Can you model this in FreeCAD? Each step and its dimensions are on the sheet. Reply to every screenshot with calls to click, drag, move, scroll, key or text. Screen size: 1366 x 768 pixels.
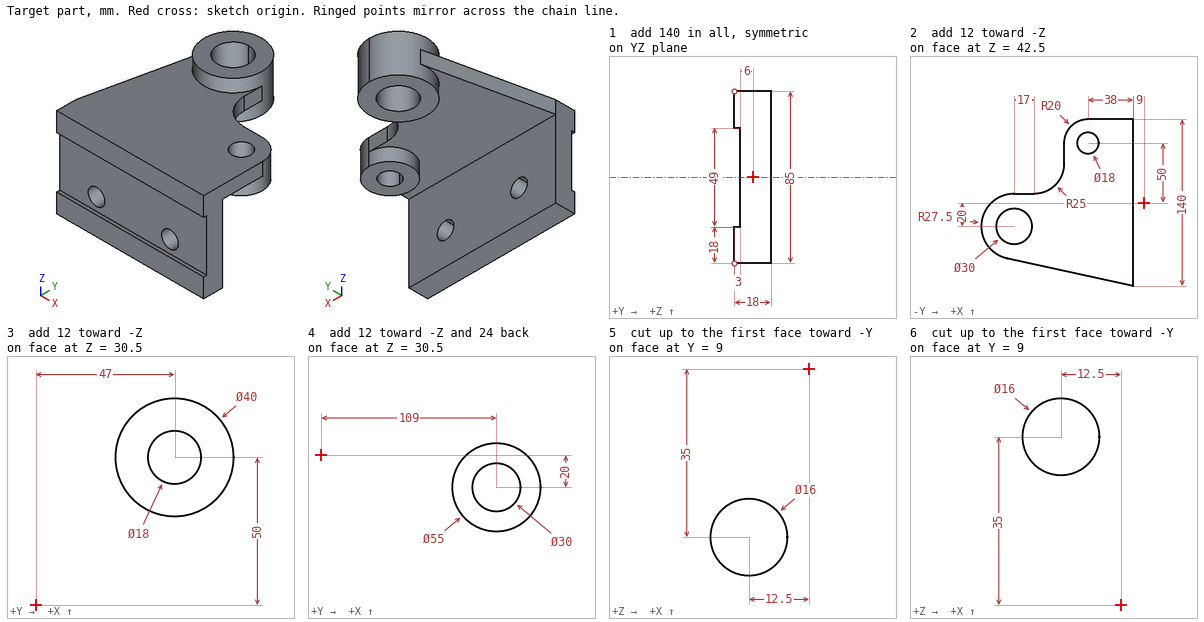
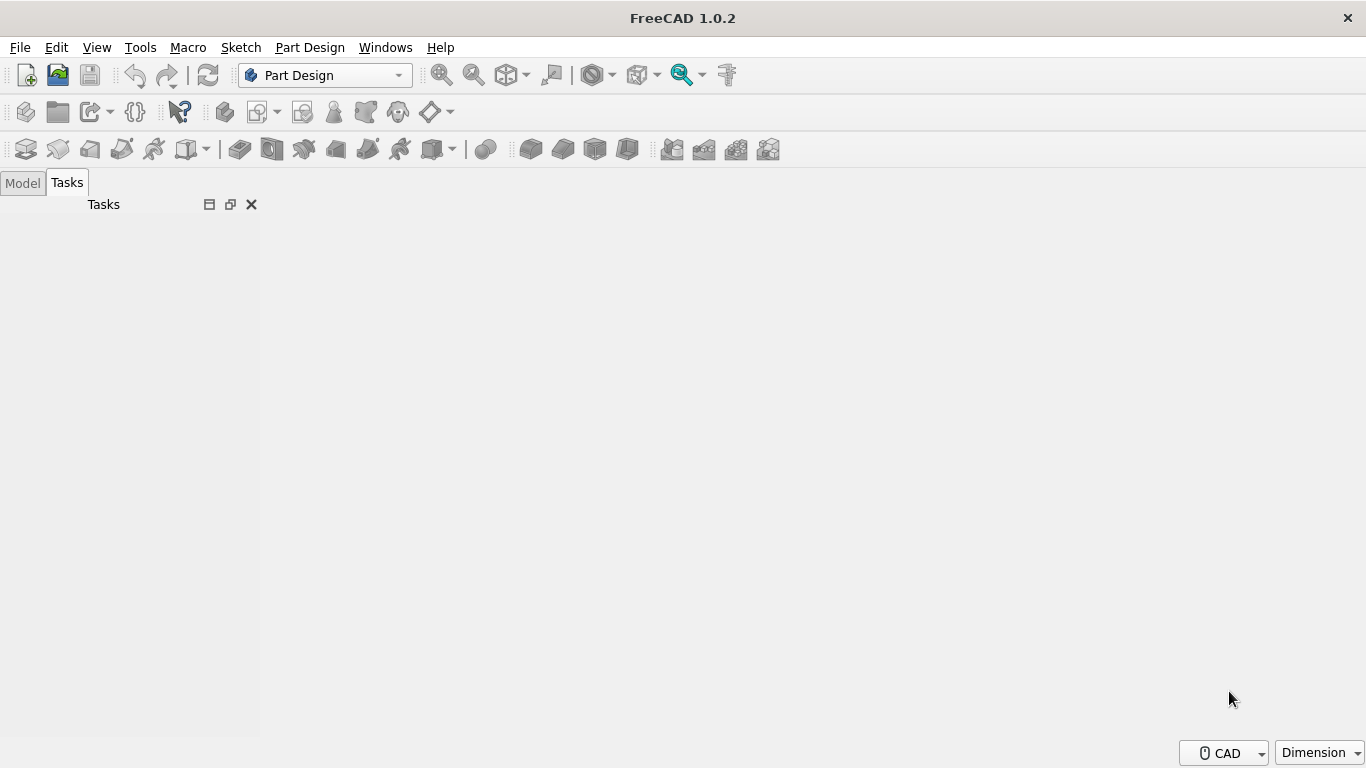
key(ctrl+n)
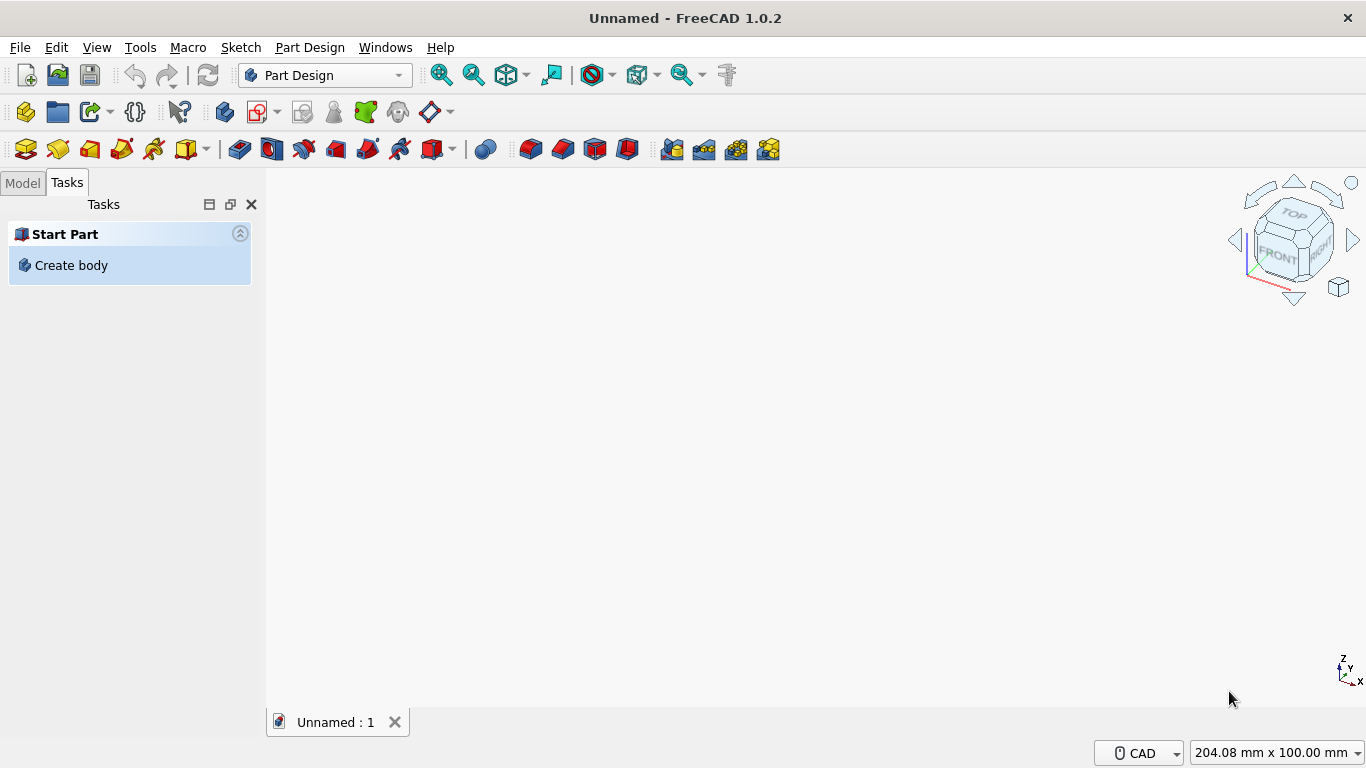
click(258, 112)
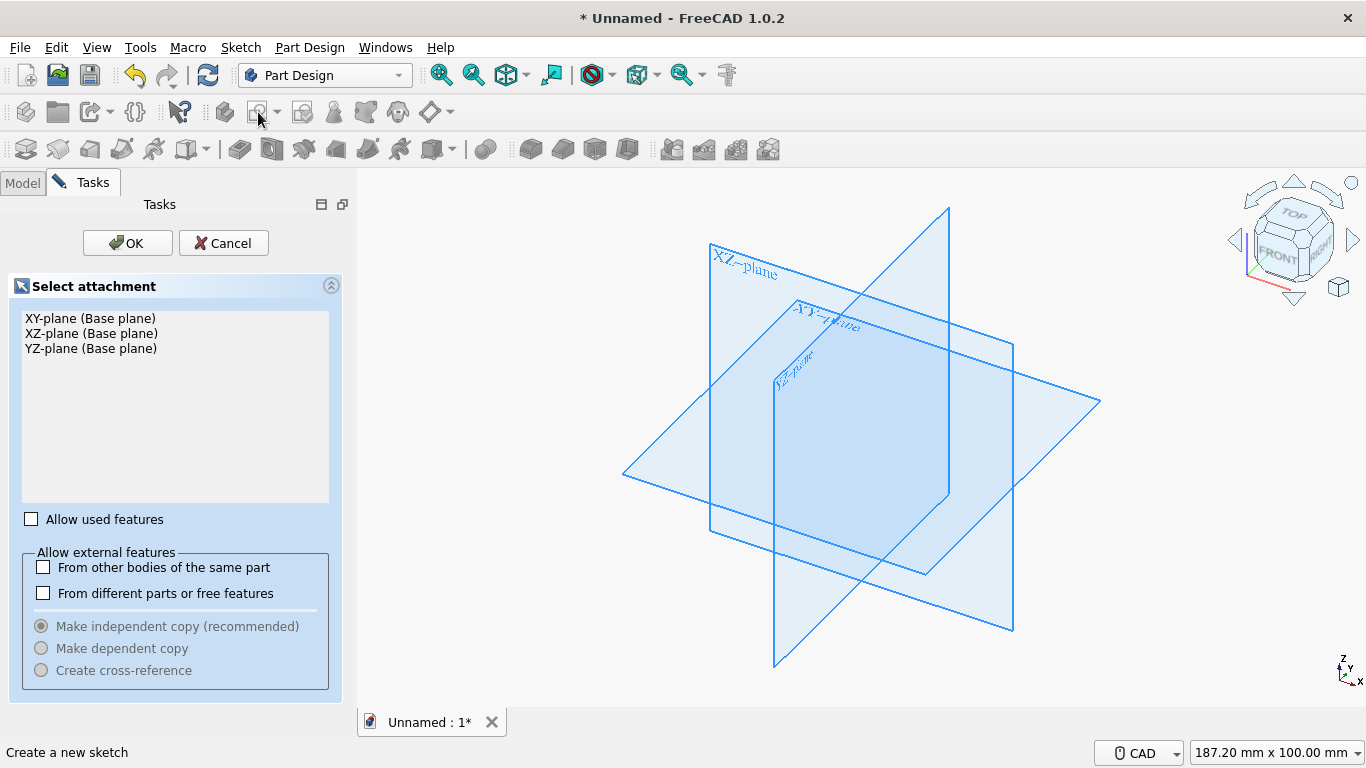
click(82, 348)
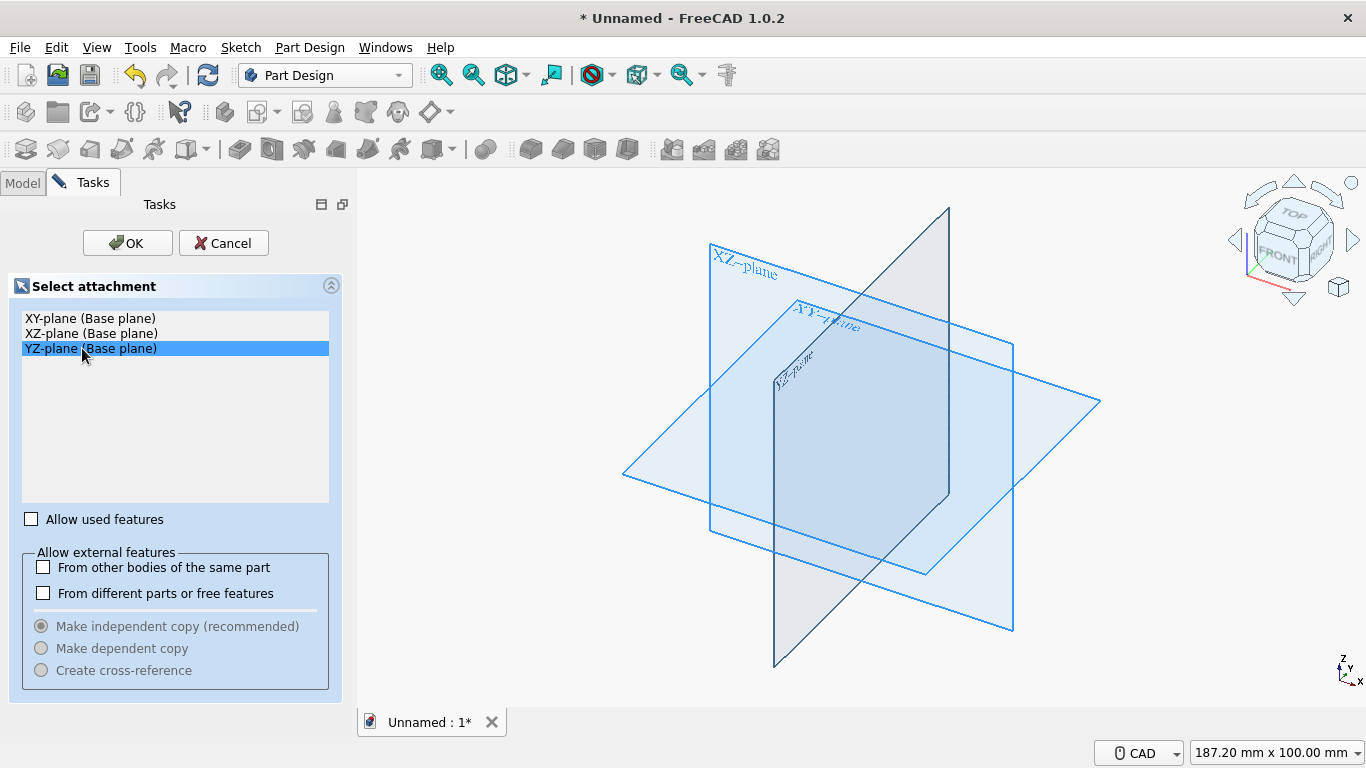
click(128, 243)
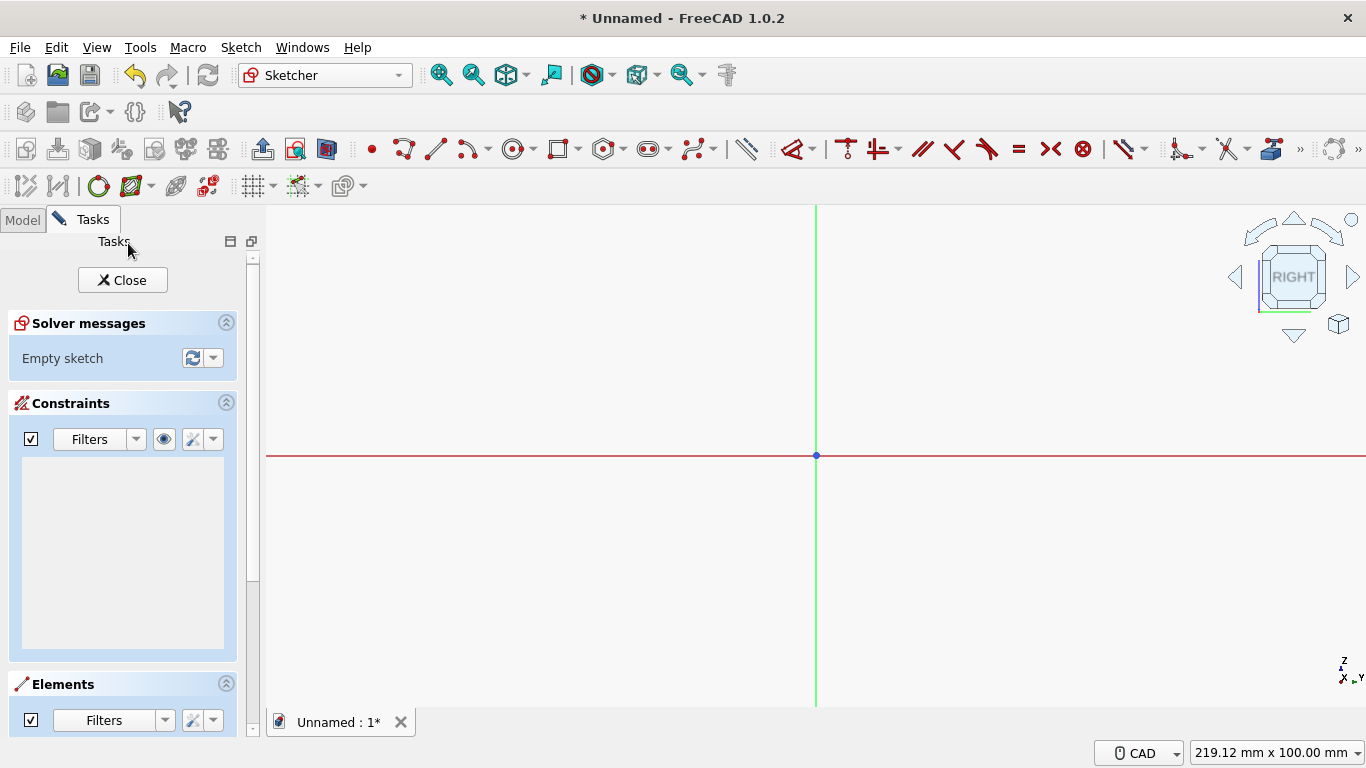
scroll(608, 456, down, 2)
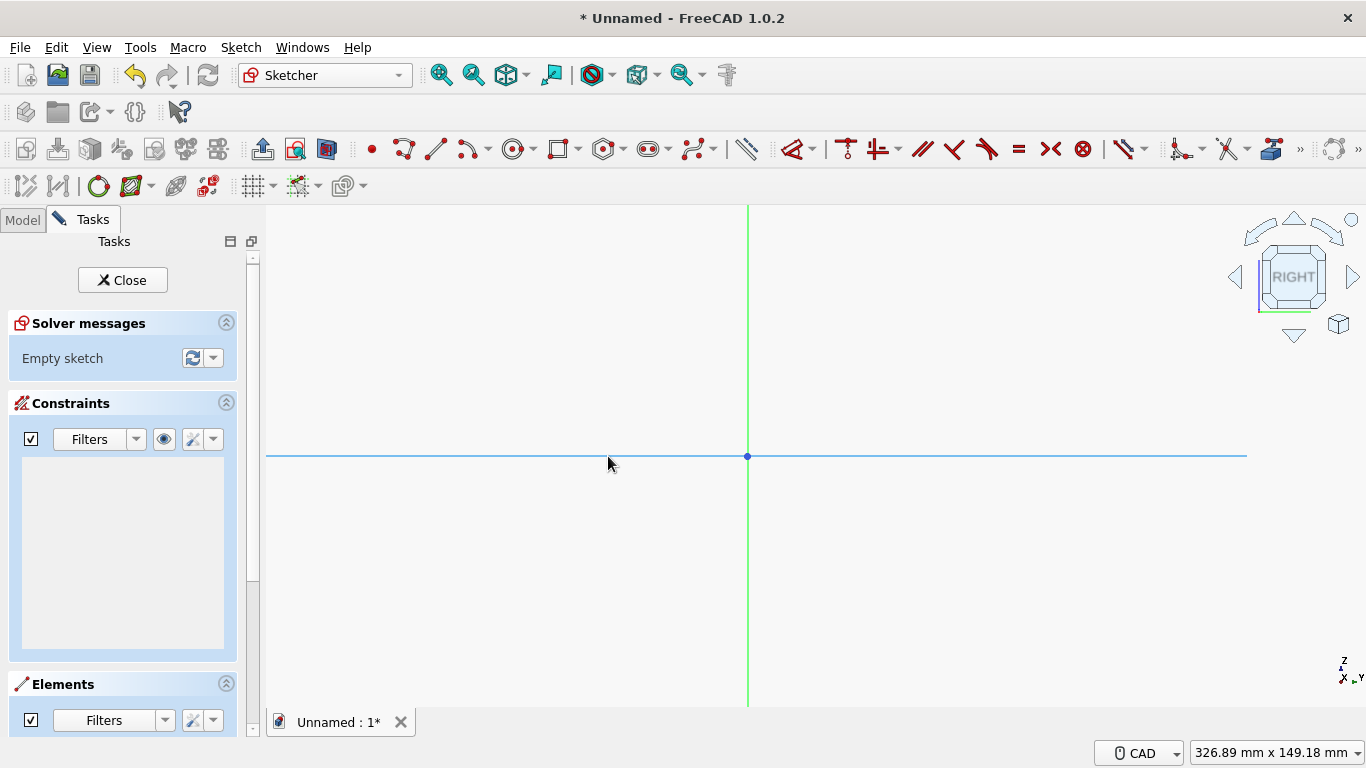
key(g)
key(m)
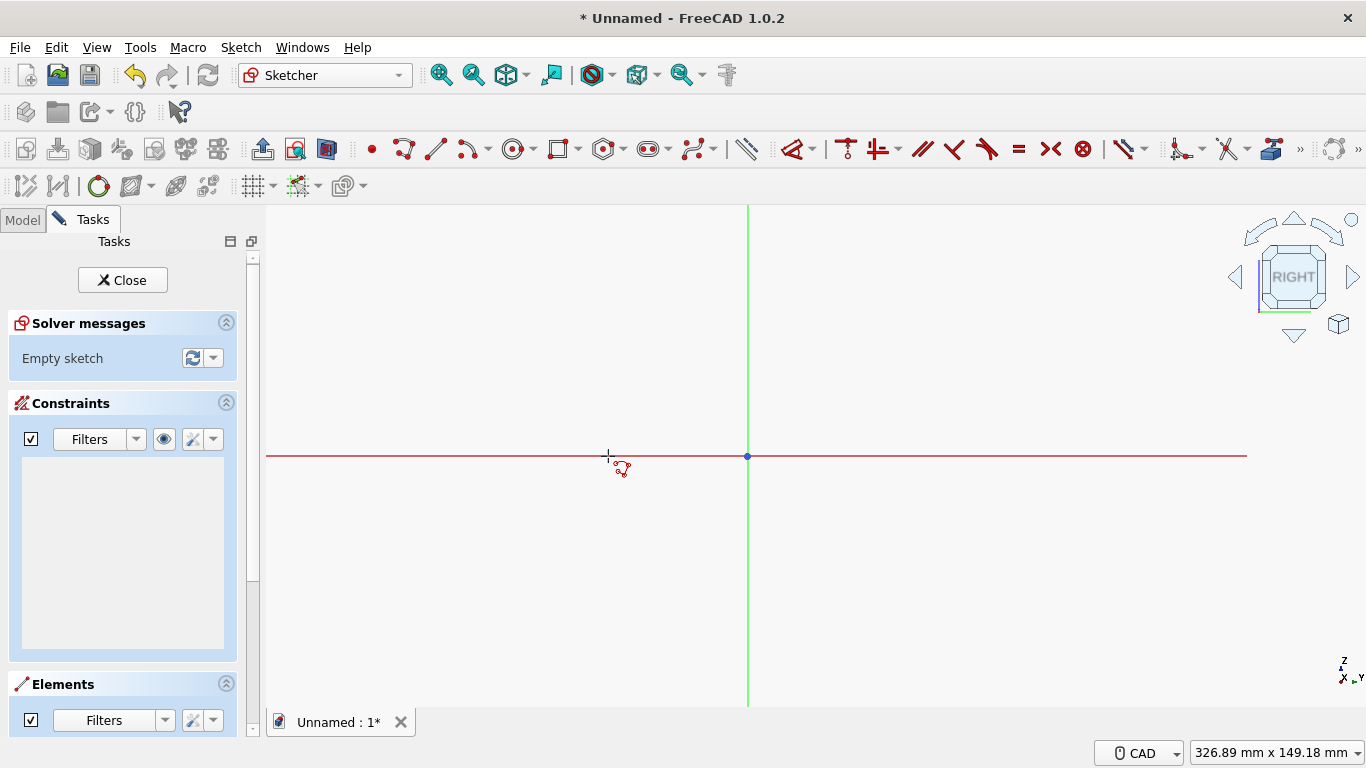
click(727, 374)
click(727, 539)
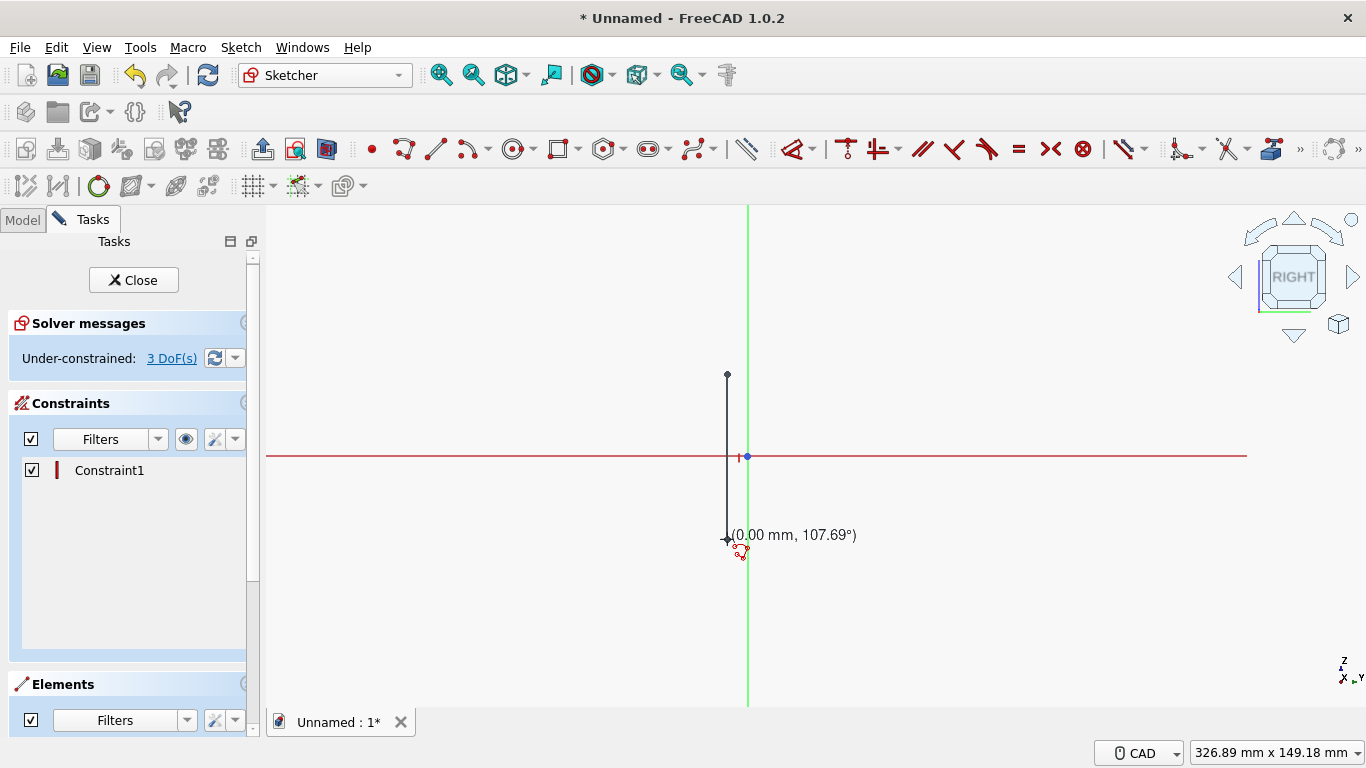
scroll(717, 539, up, 3)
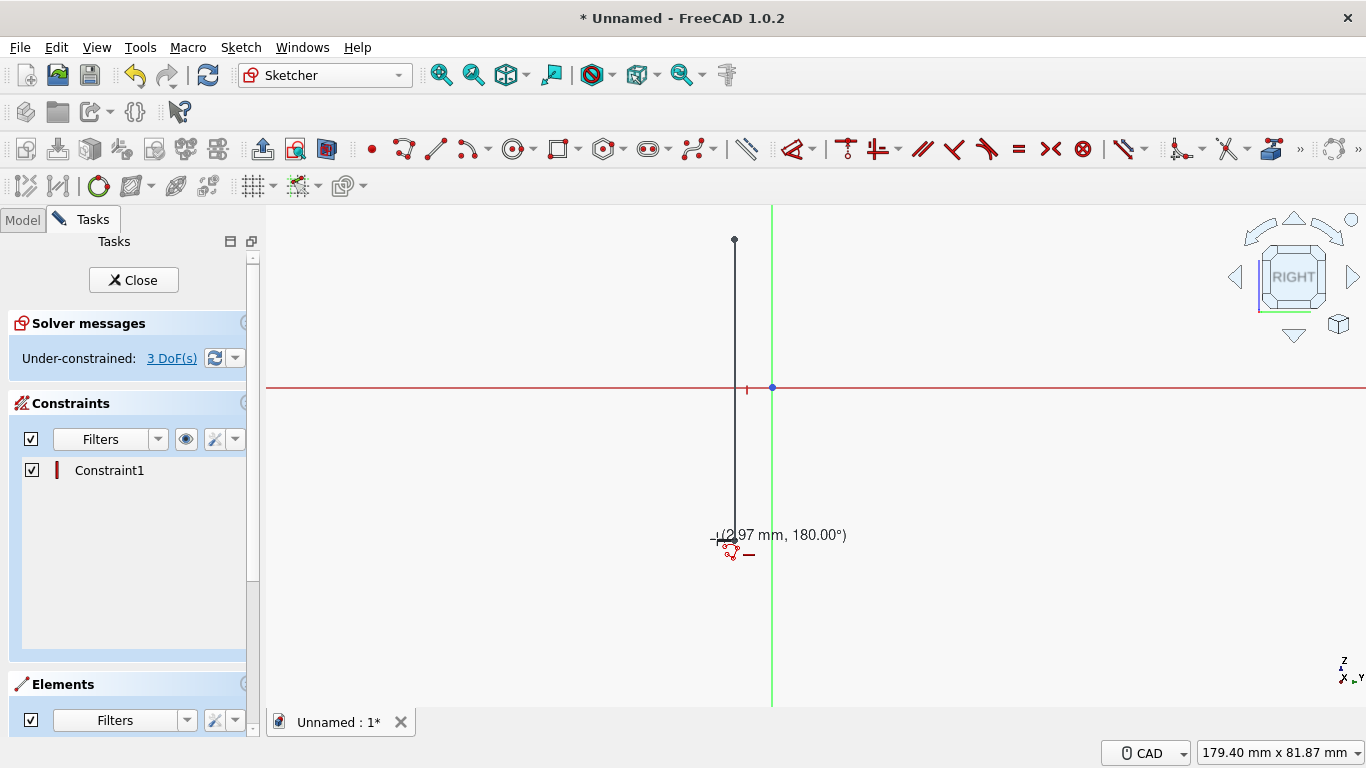
click(717, 538)
click(717, 648)
click(827, 648)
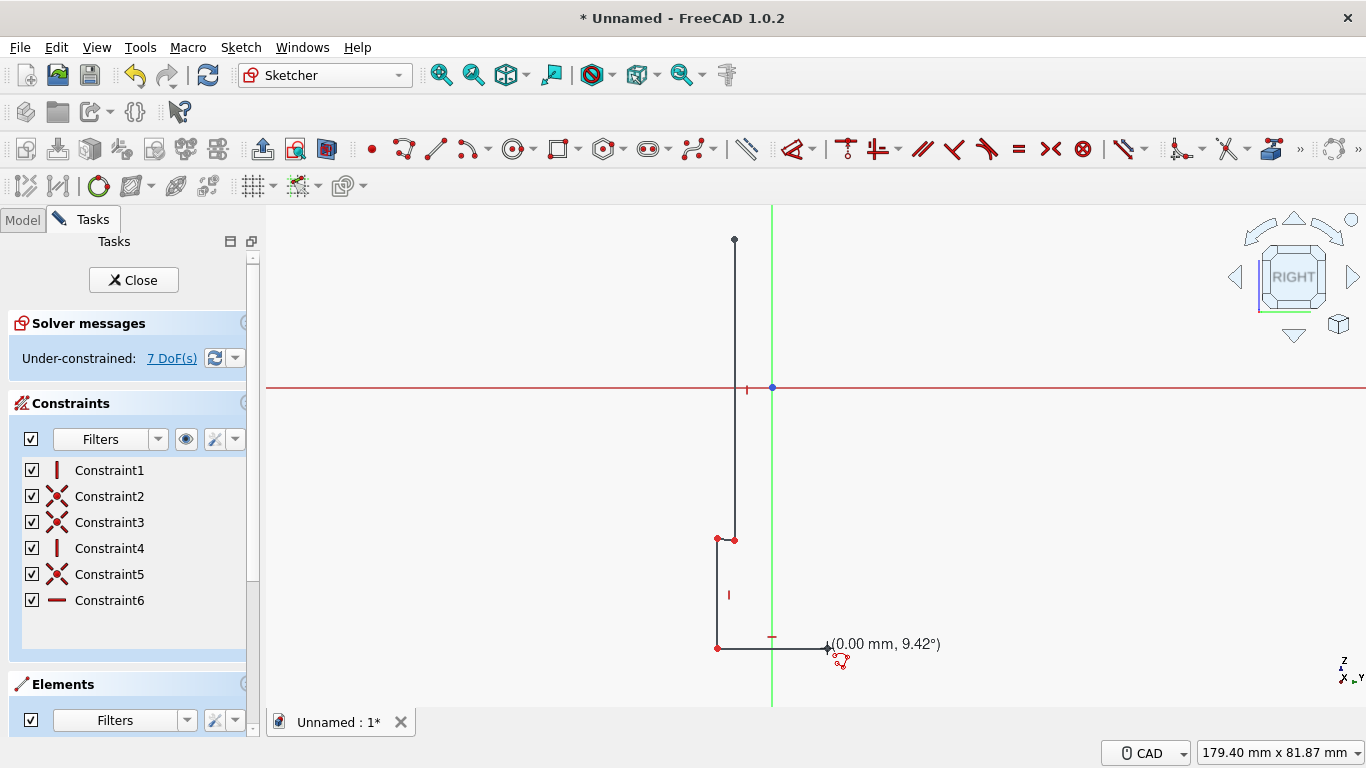
scroll(717, 539, down, 3)